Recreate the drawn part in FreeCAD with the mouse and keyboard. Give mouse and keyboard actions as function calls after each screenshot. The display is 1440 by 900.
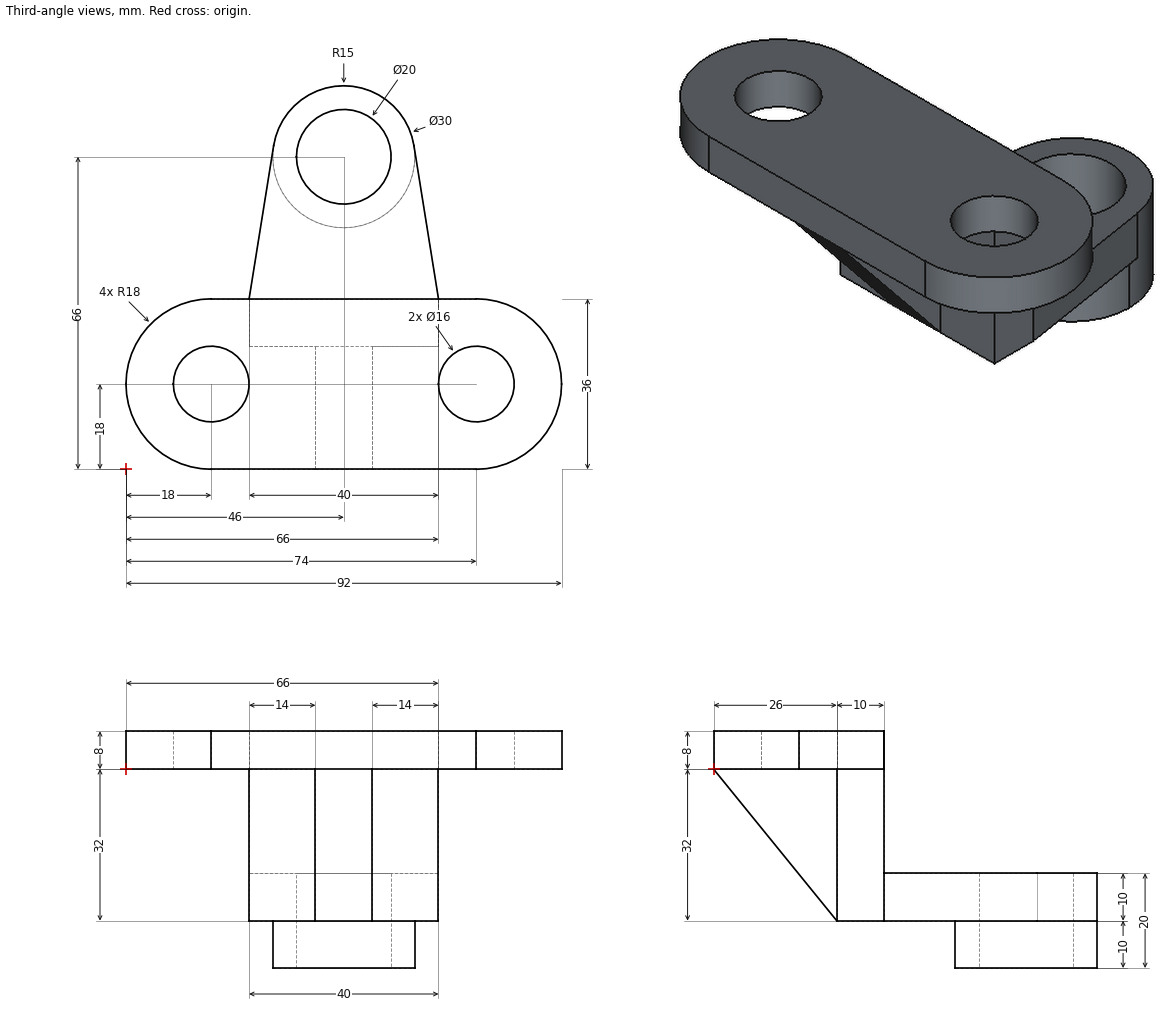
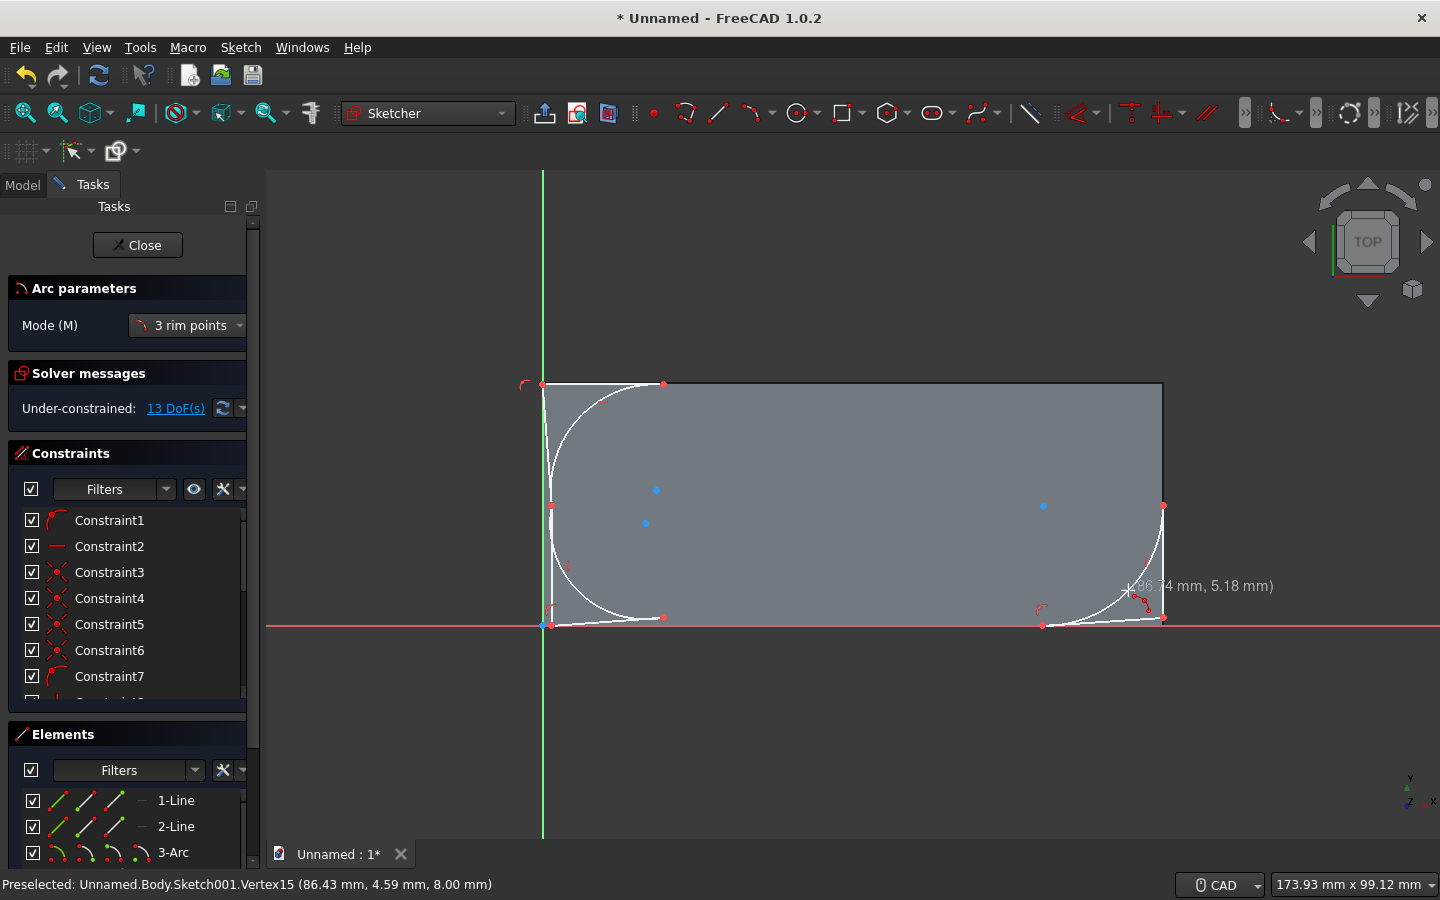
click(686, 114)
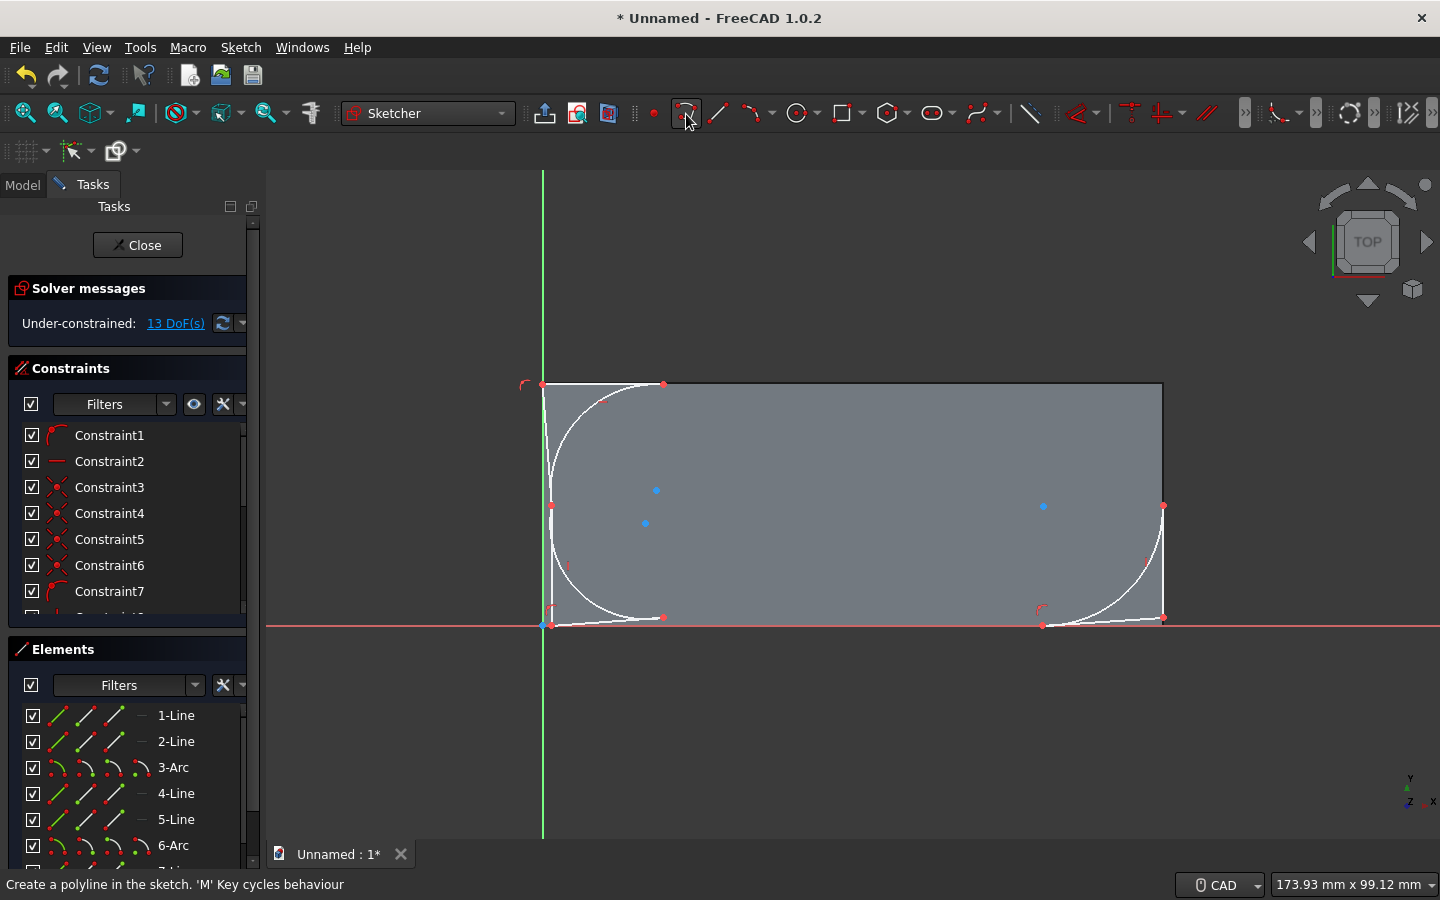
click(1163, 506)
click(1163, 383)
click(1042, 383)
right_click(1042, 383)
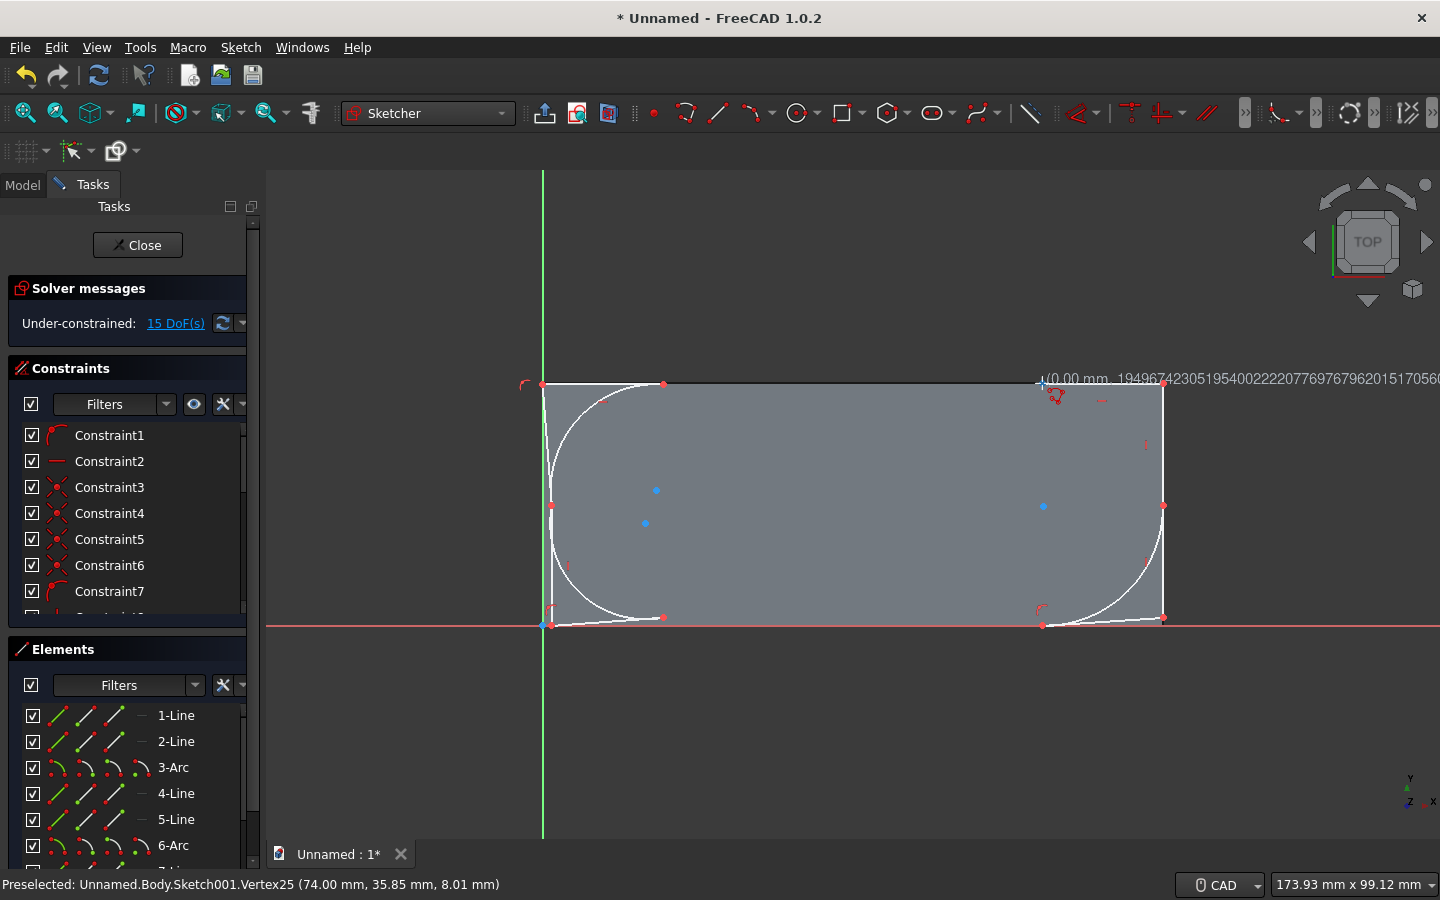
click(752, 114)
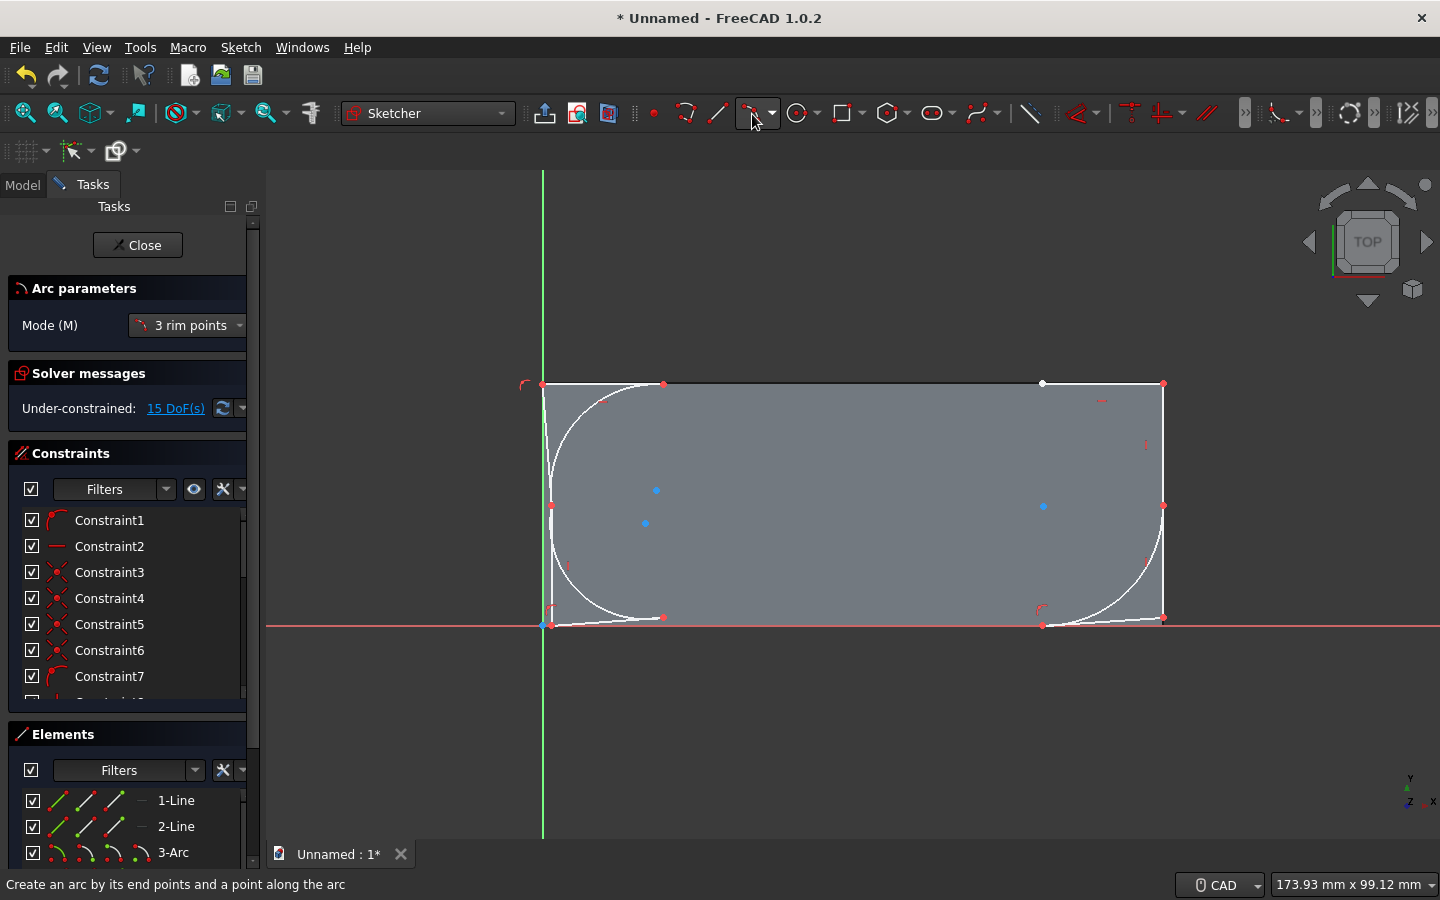
click(1042, 384)
click(1163, 506)
click(1128, 419)
key(Escape)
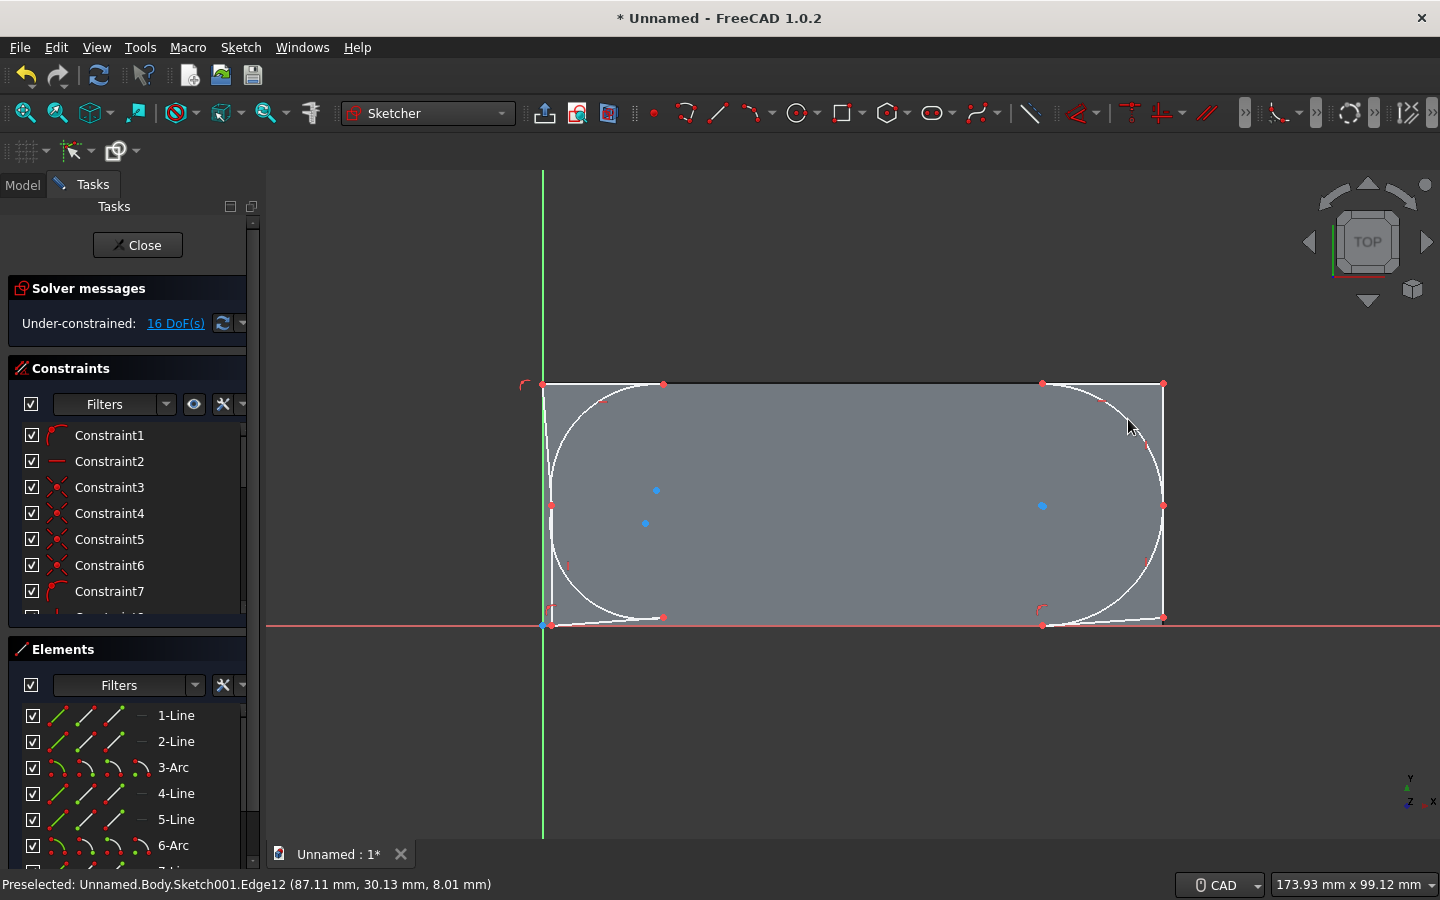
click(579, 384)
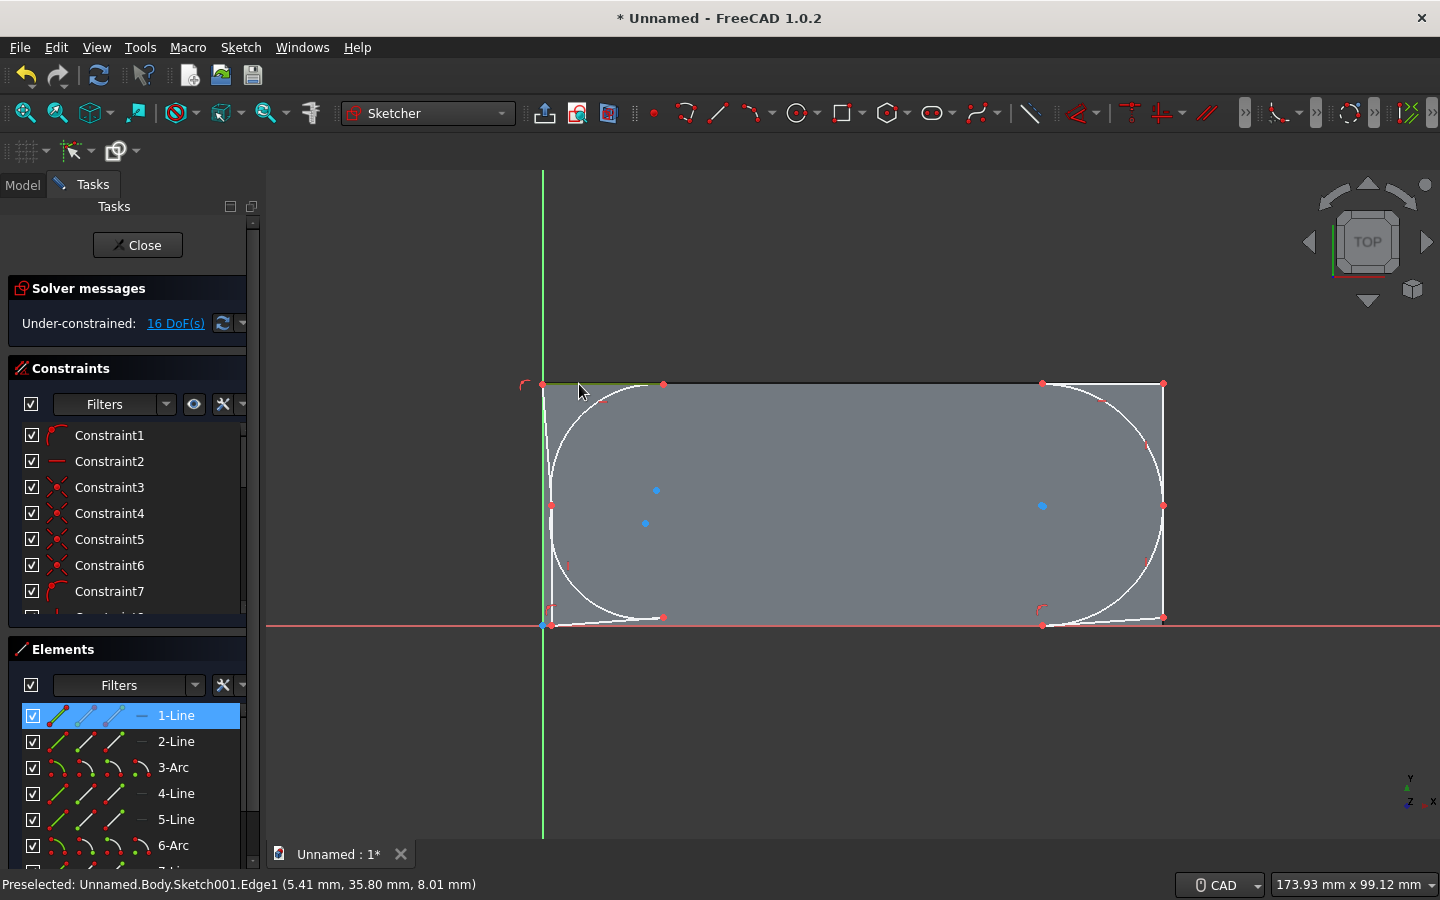
scroll(609, 396, up, 2)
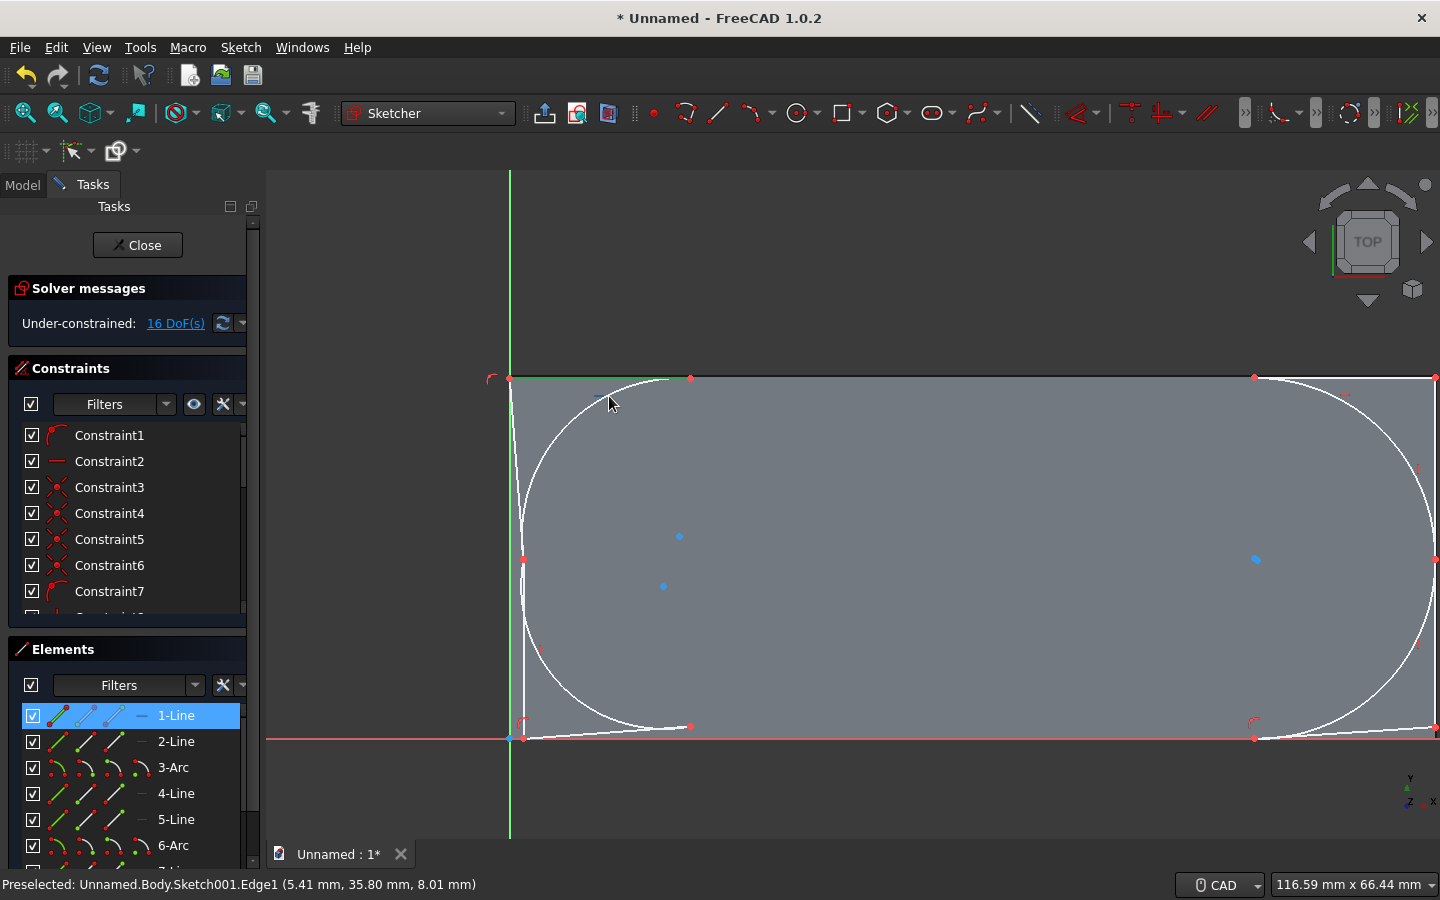
click(608, 395)